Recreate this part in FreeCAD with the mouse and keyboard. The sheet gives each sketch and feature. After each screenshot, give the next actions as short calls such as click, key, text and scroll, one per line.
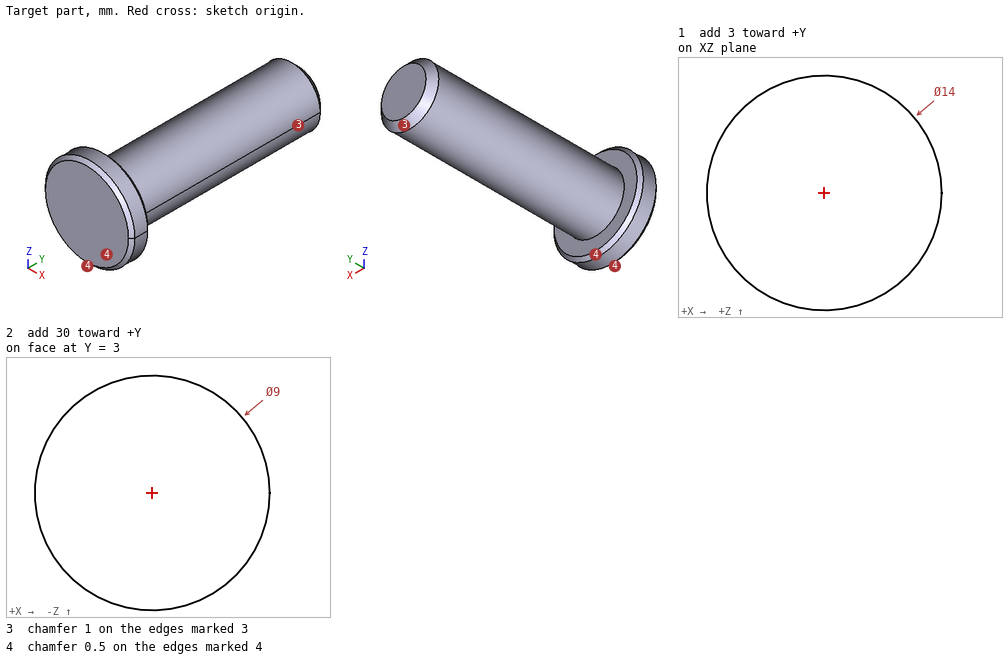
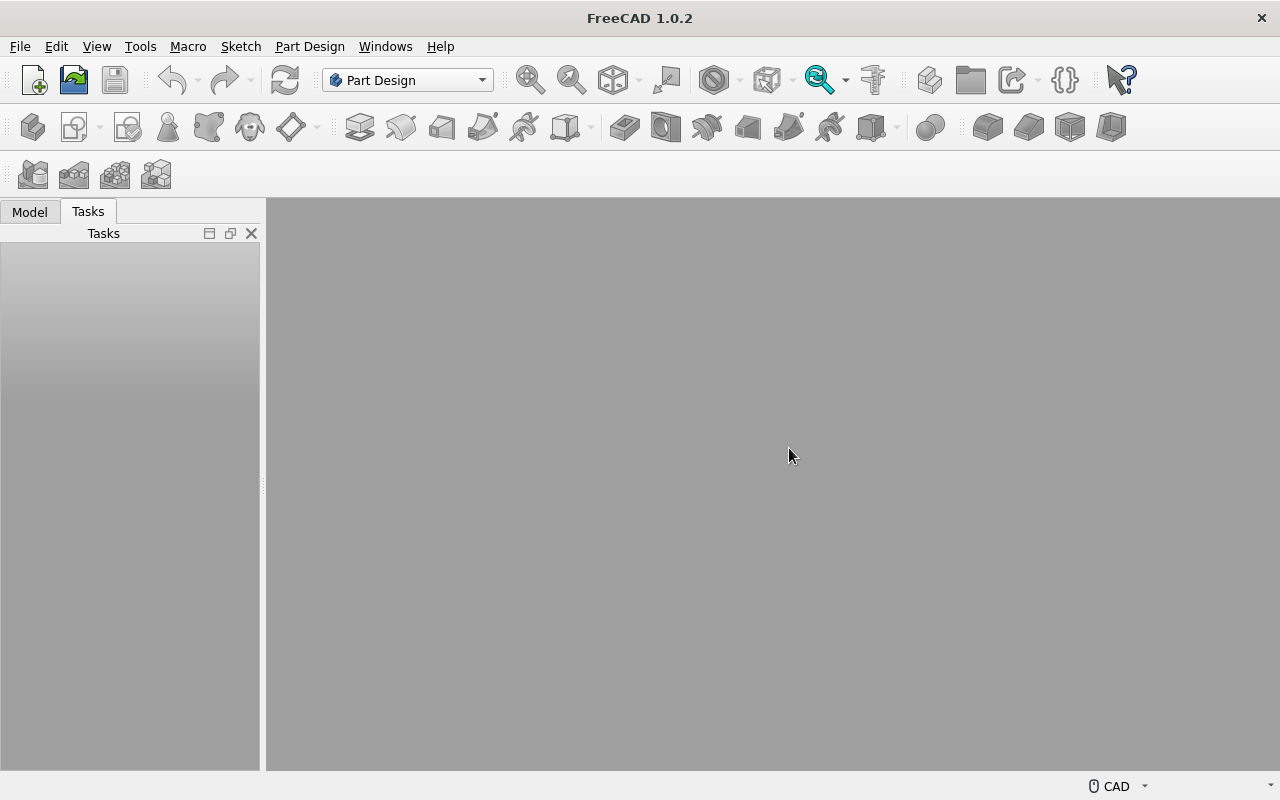
key(ctrl+n)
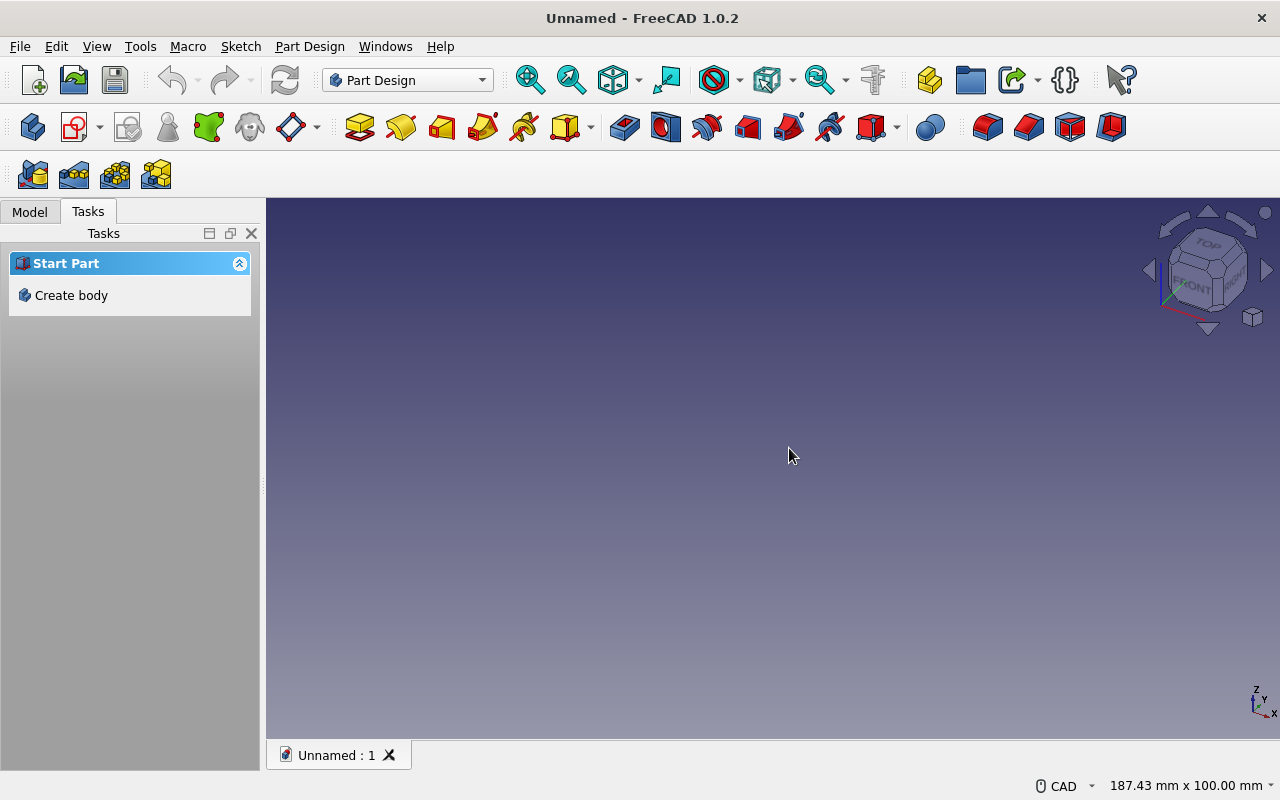
click(74, 128)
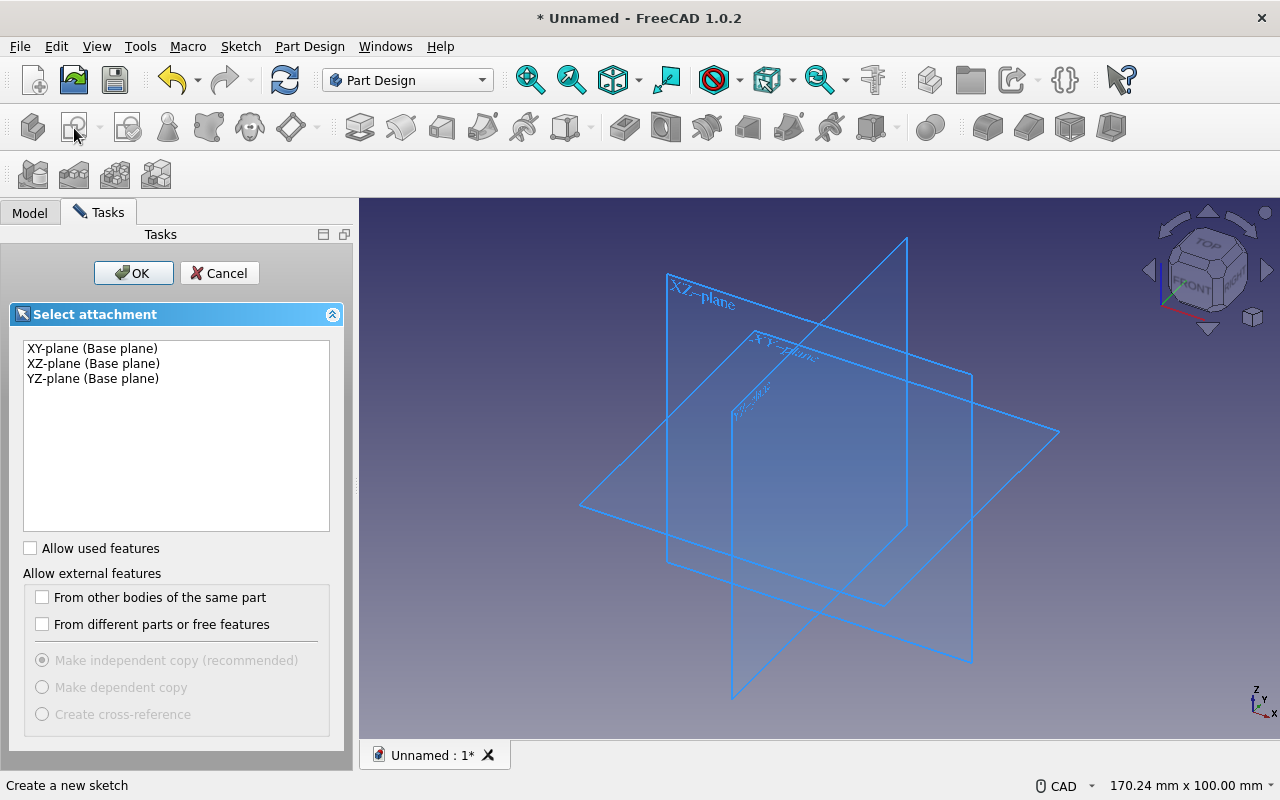
click(84, 364)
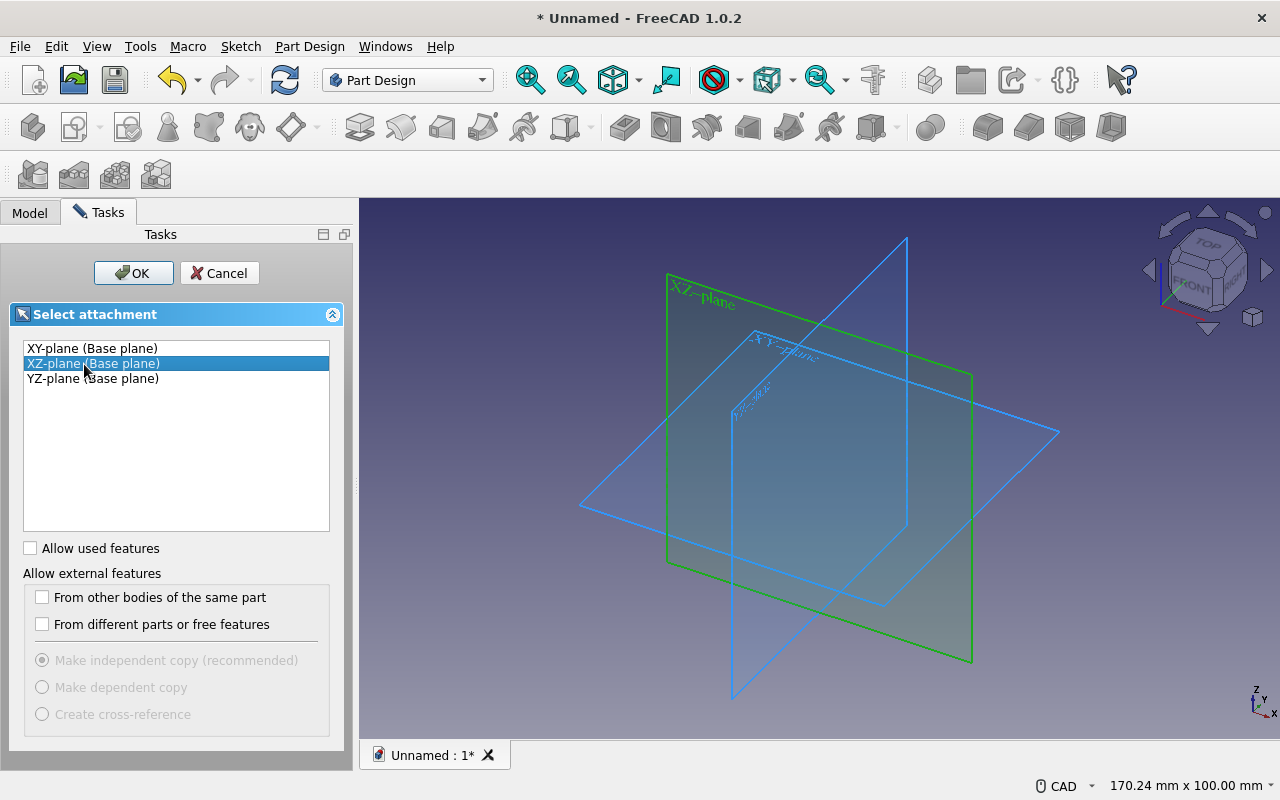
click(134, 273)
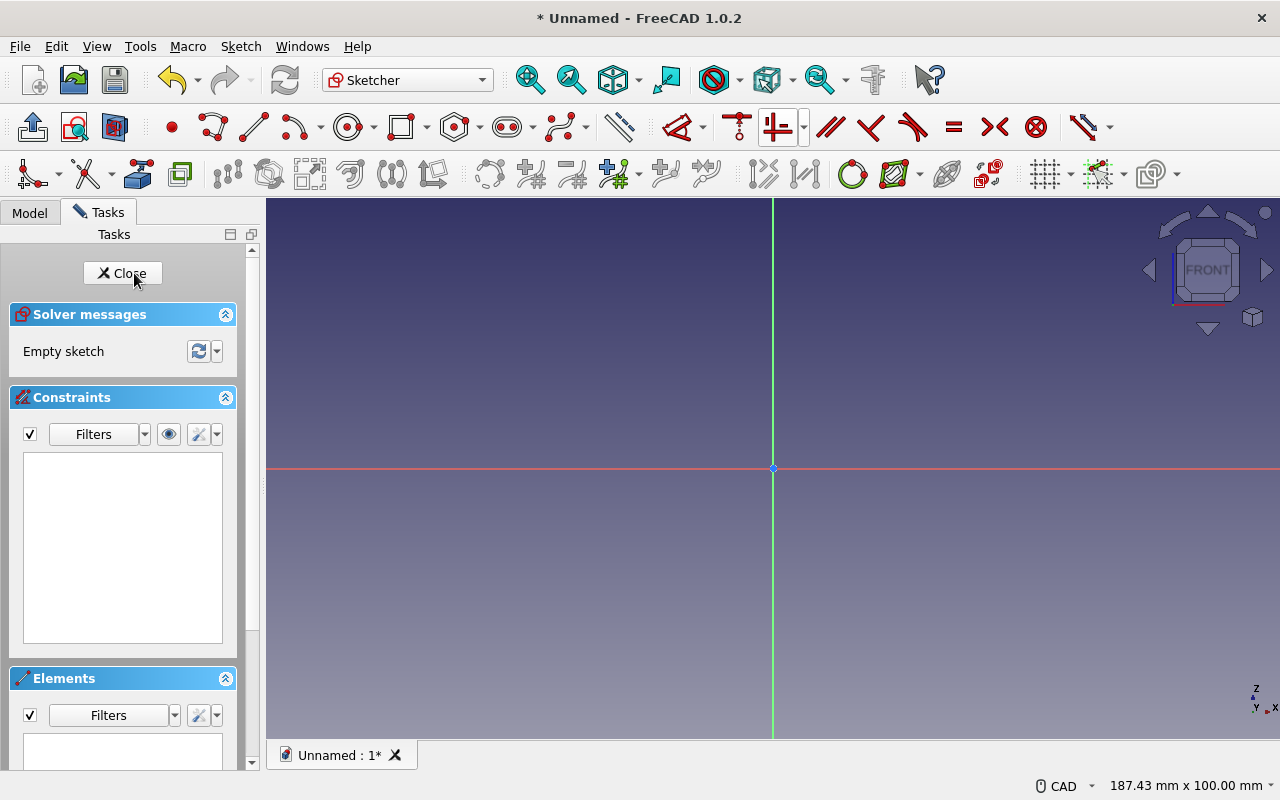
scroll(790, 469, up, 8)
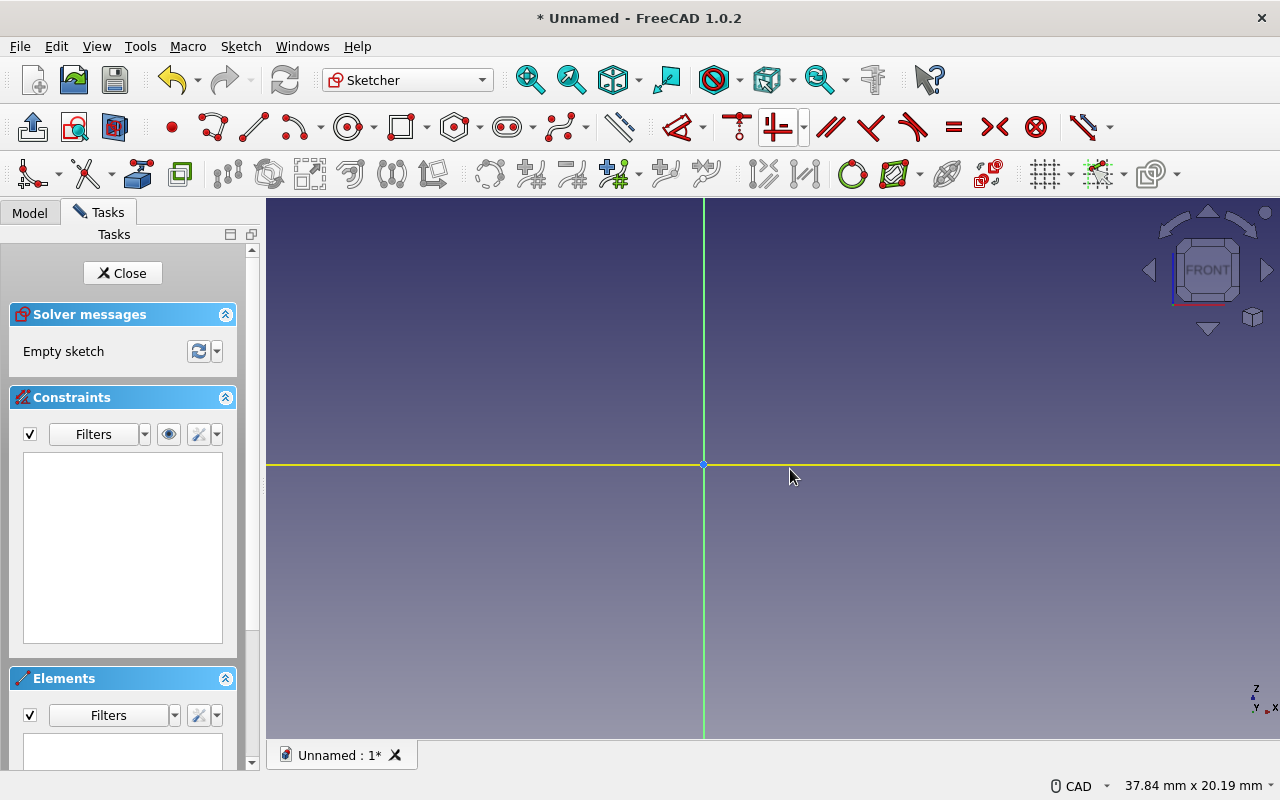
key(g)
key(c)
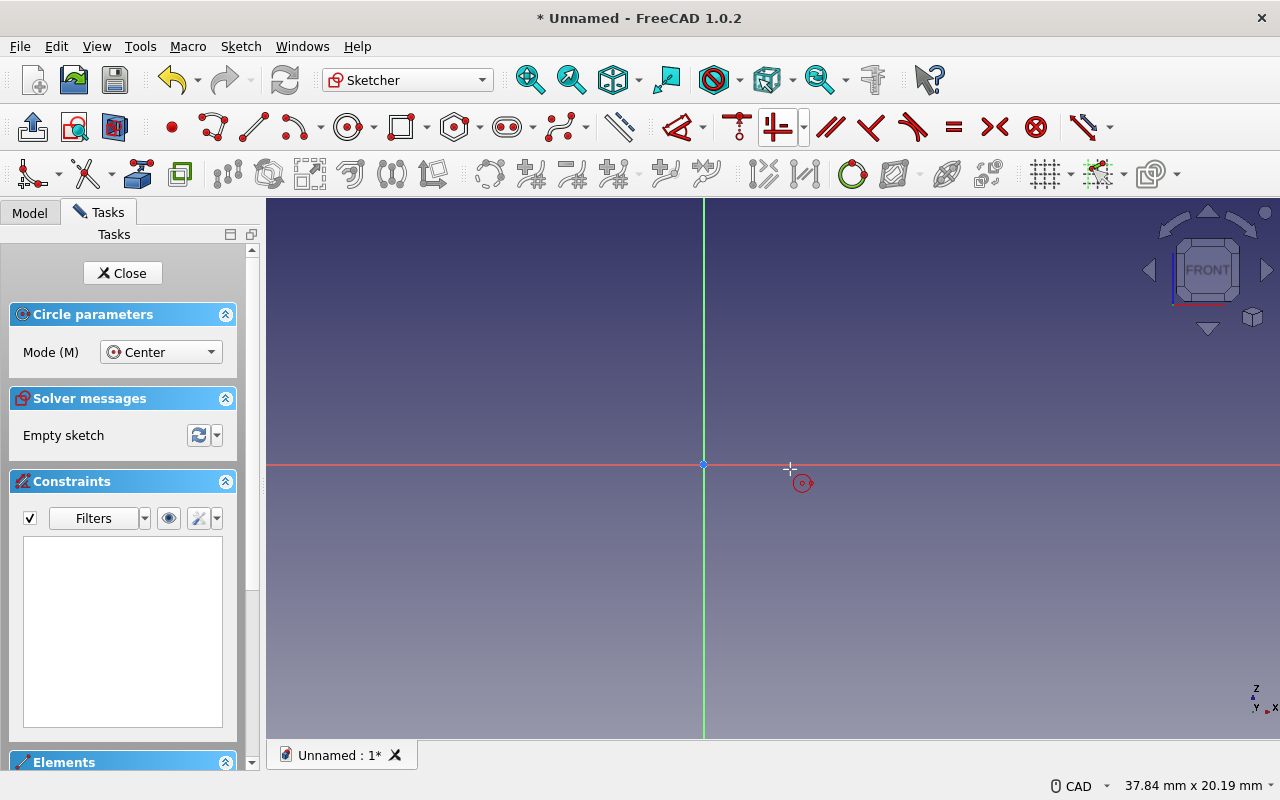
click(704, 465)
move(836, 332)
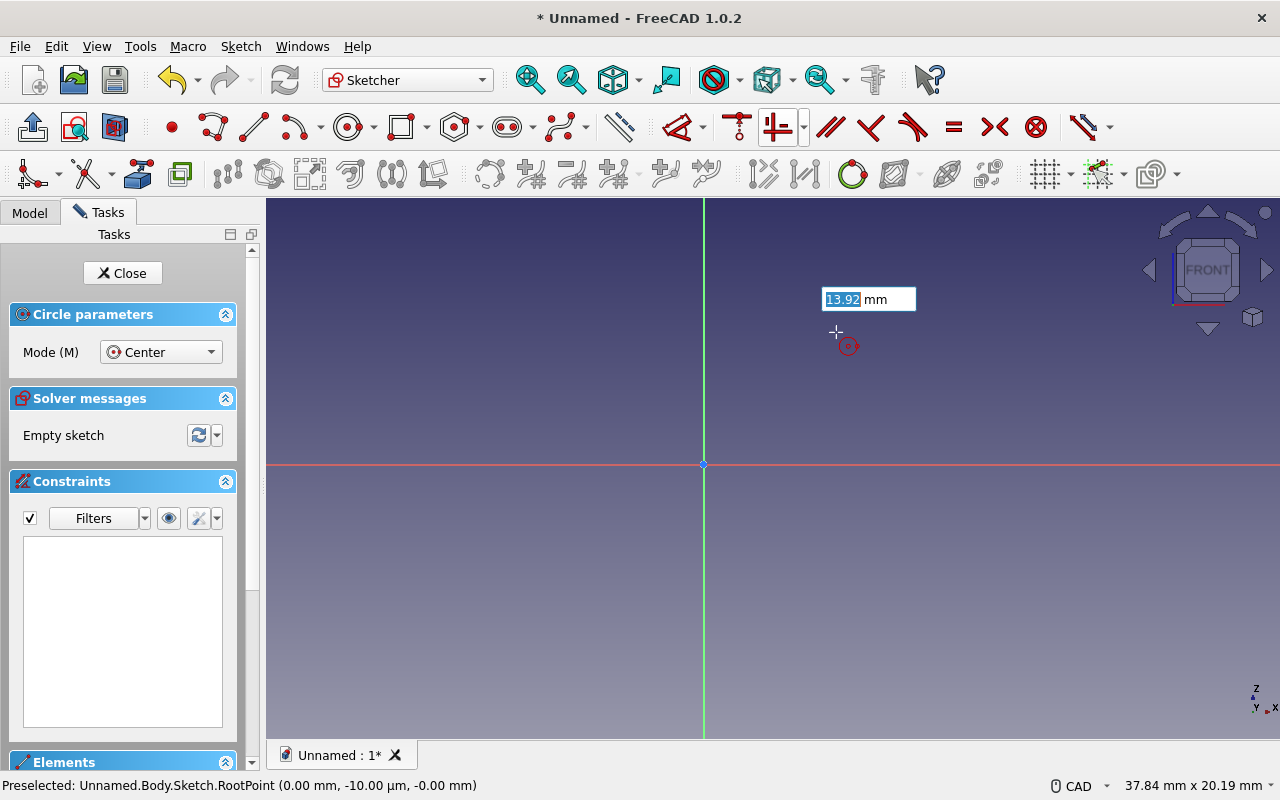
text(14)
key(Return)
key(Escape)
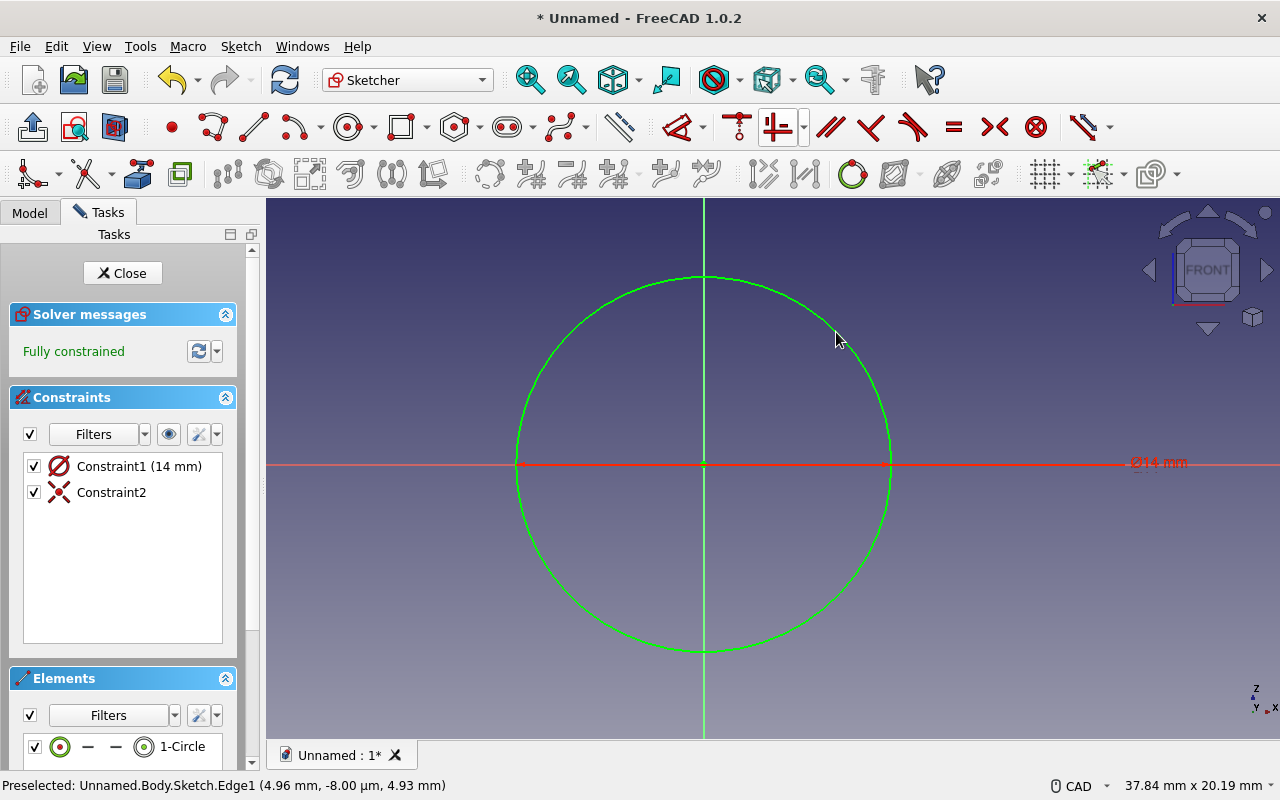
click(123, 273)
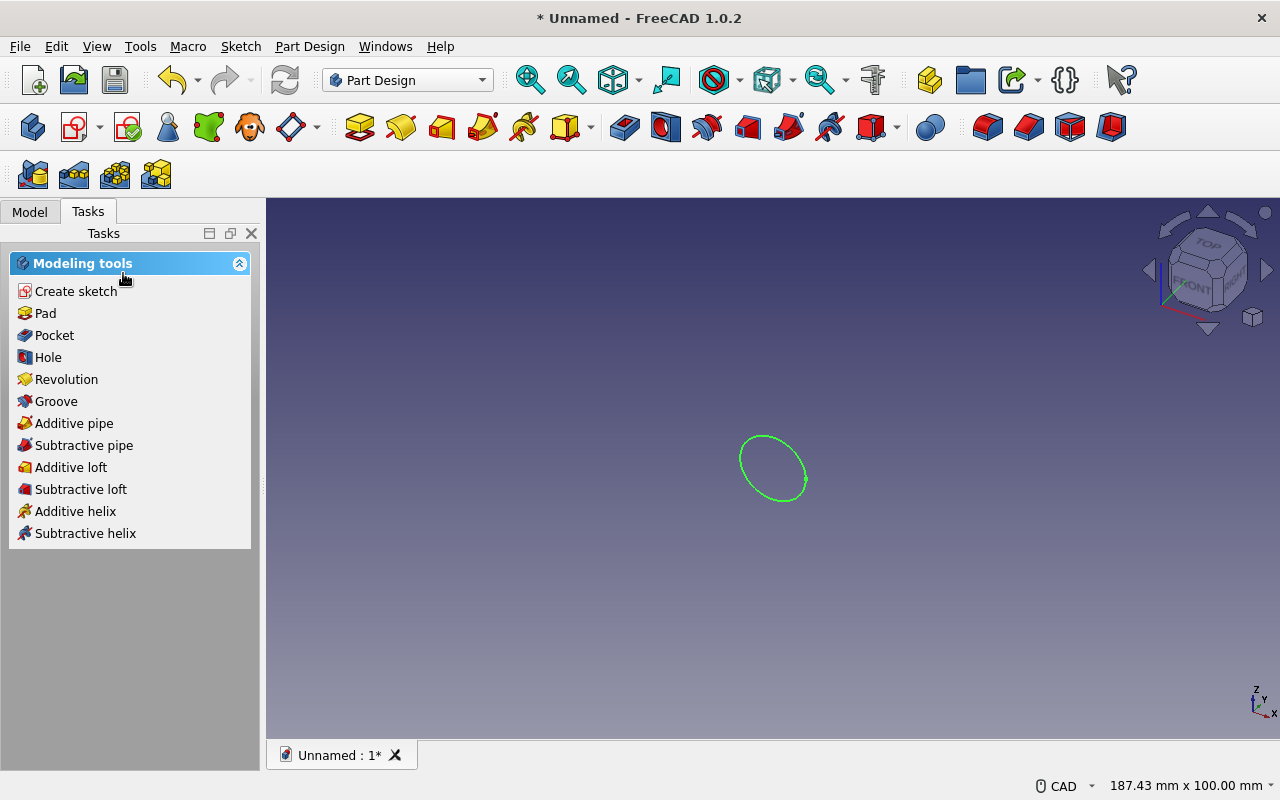
click(360, 128)